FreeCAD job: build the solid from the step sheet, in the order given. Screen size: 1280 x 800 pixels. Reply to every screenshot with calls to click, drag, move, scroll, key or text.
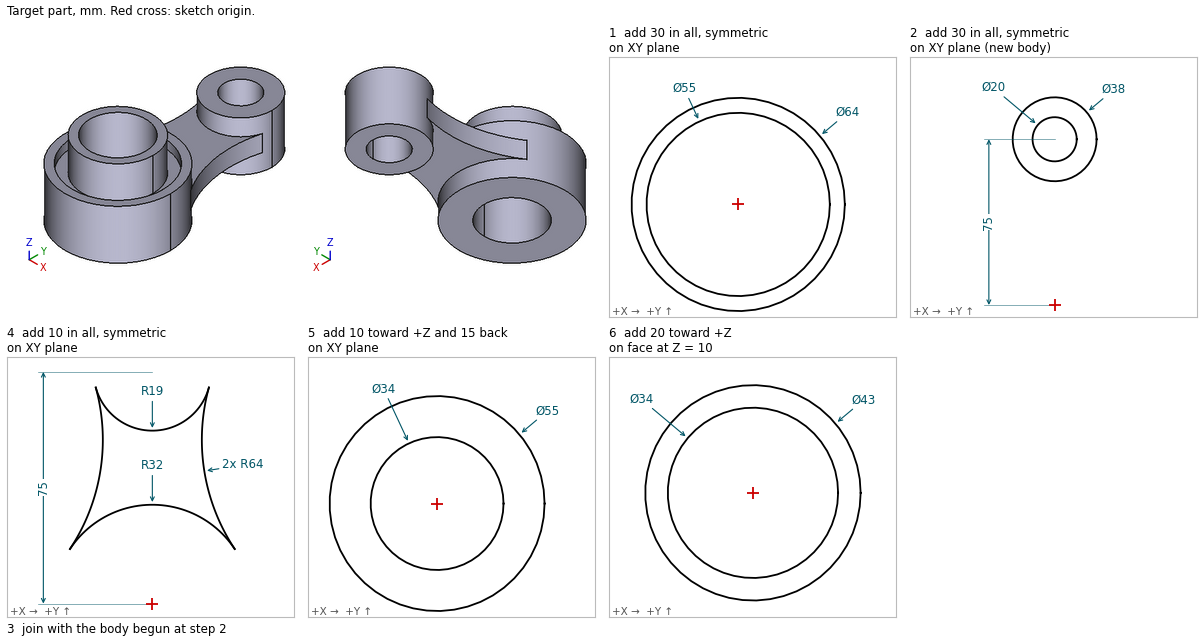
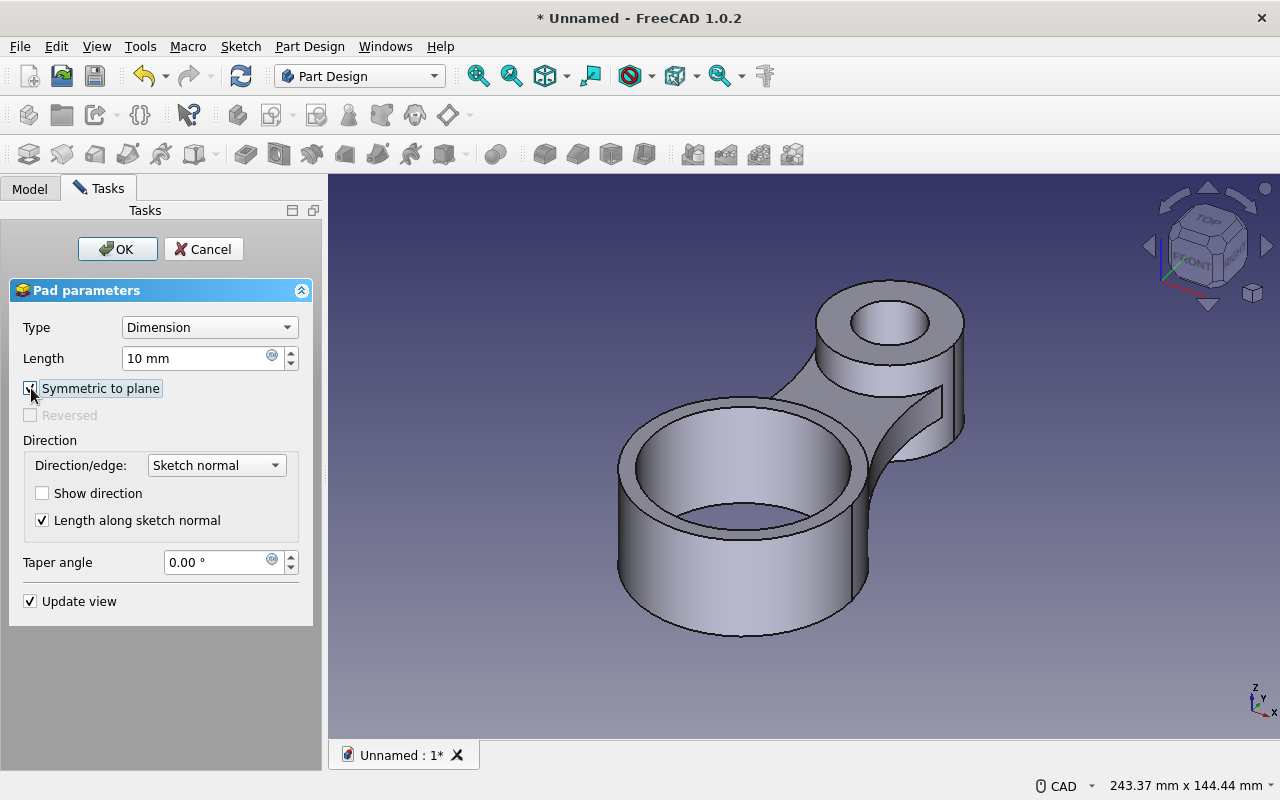
click(118, 249)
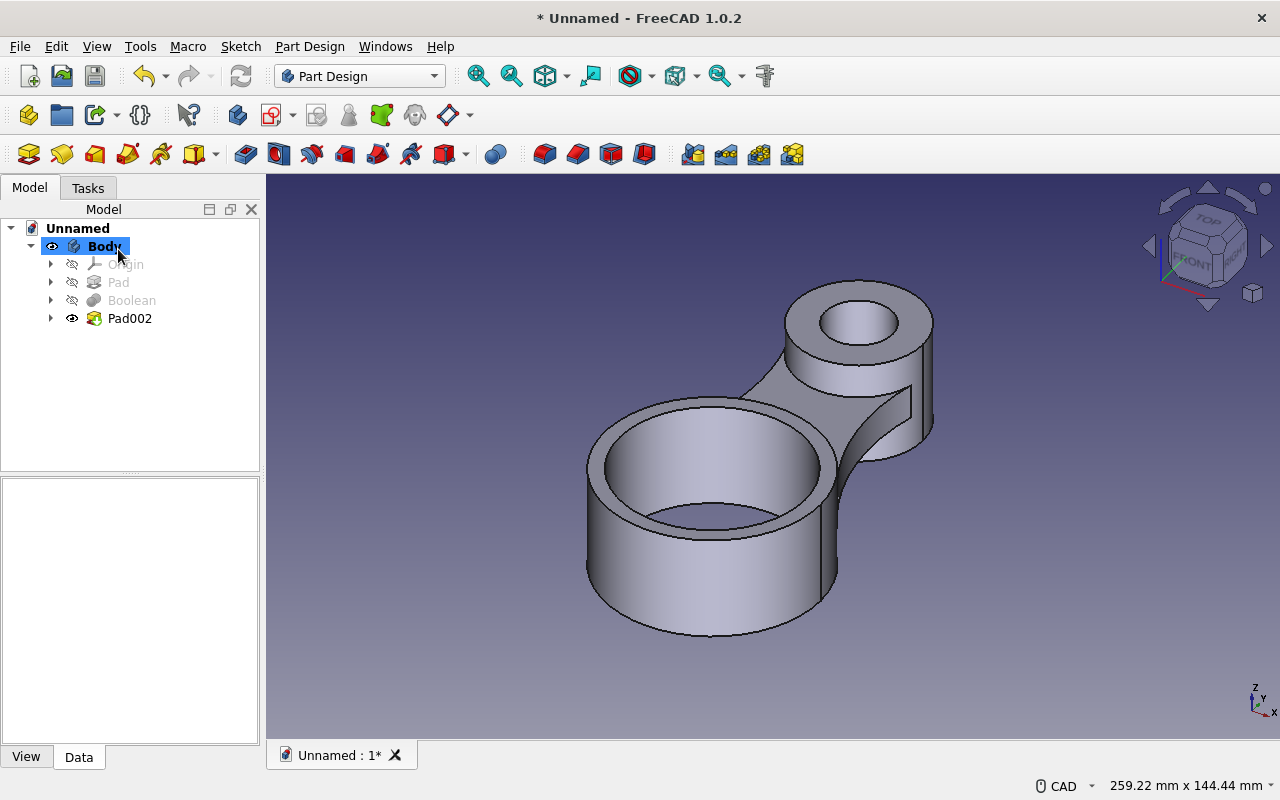
click(270, 116)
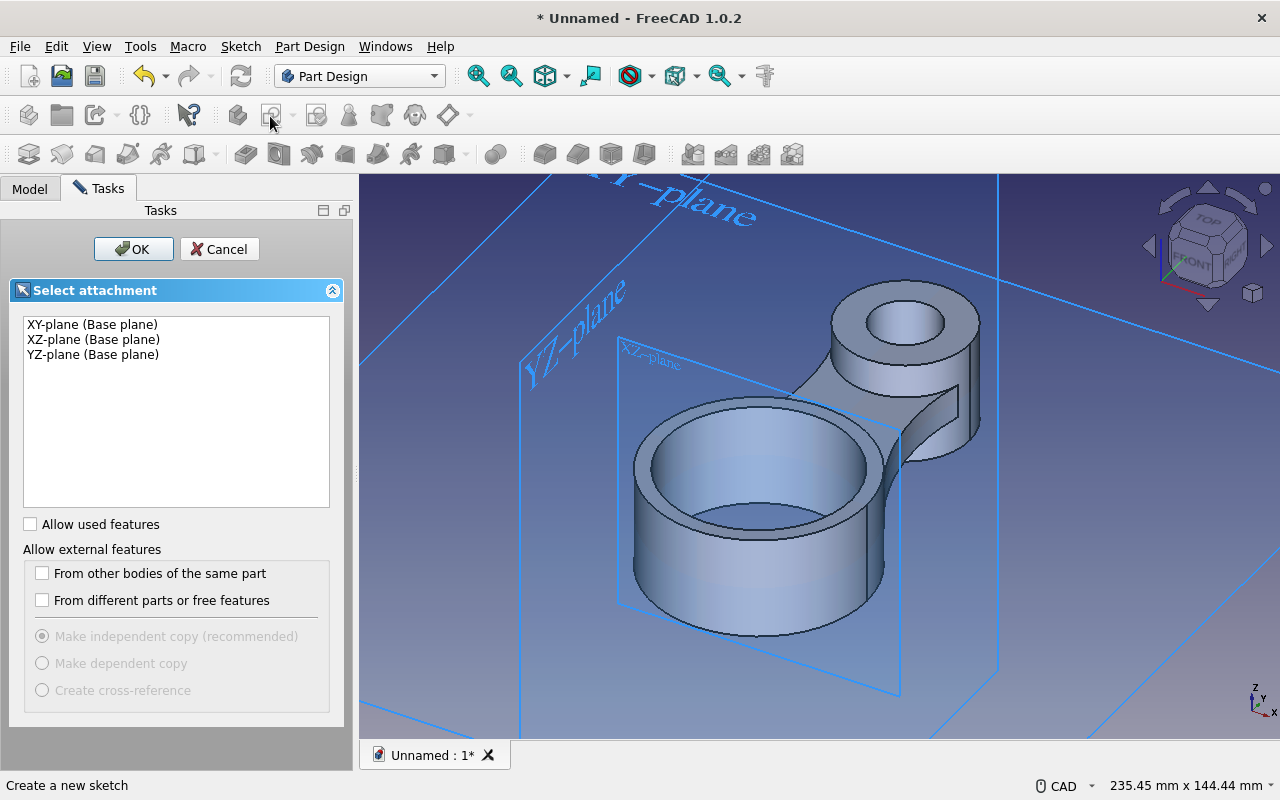
click(84, 324)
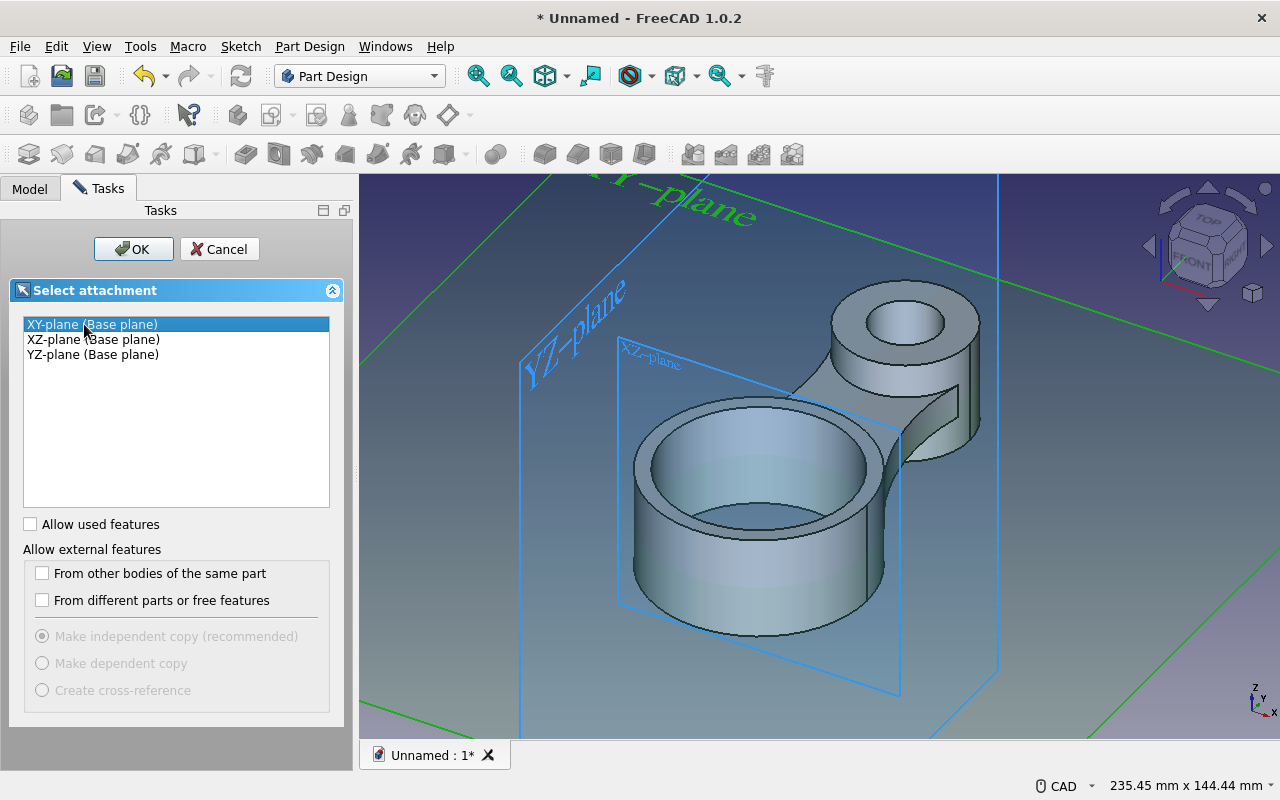
click(134, 249)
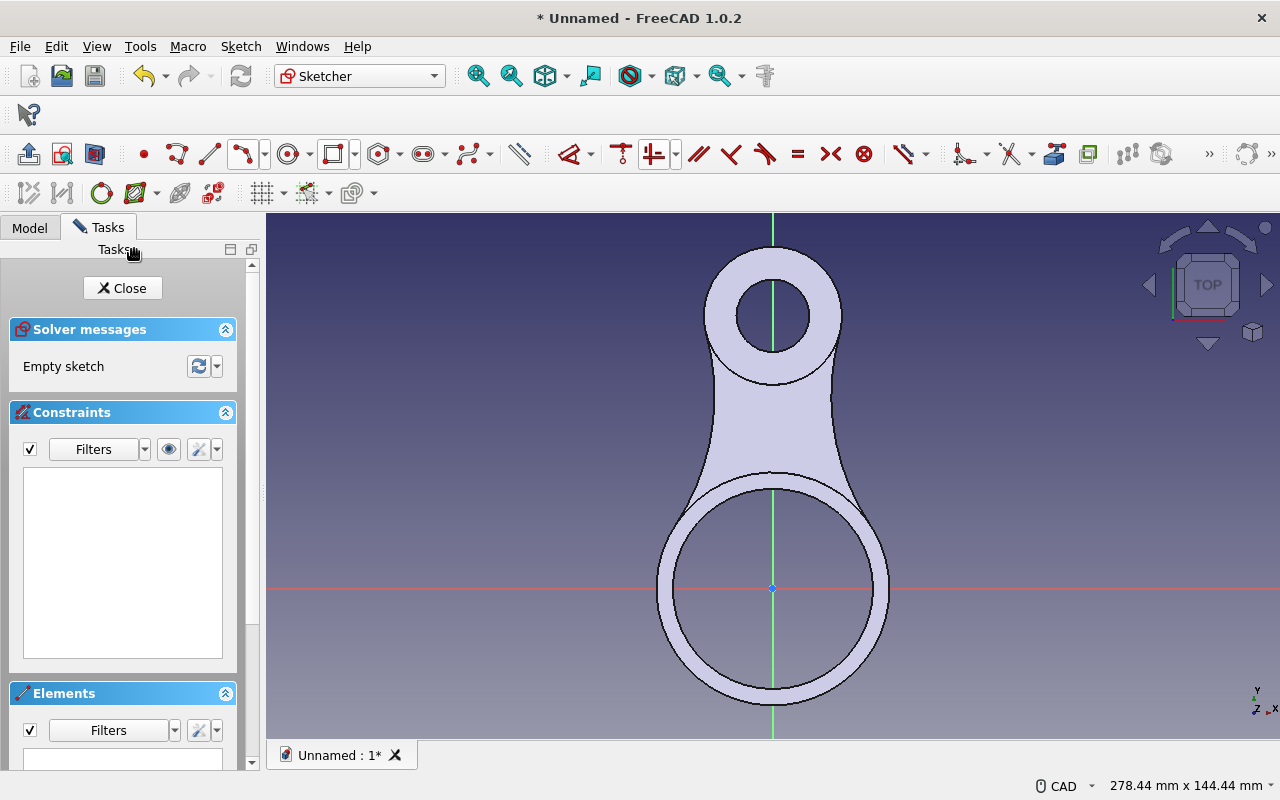
click(95, 154)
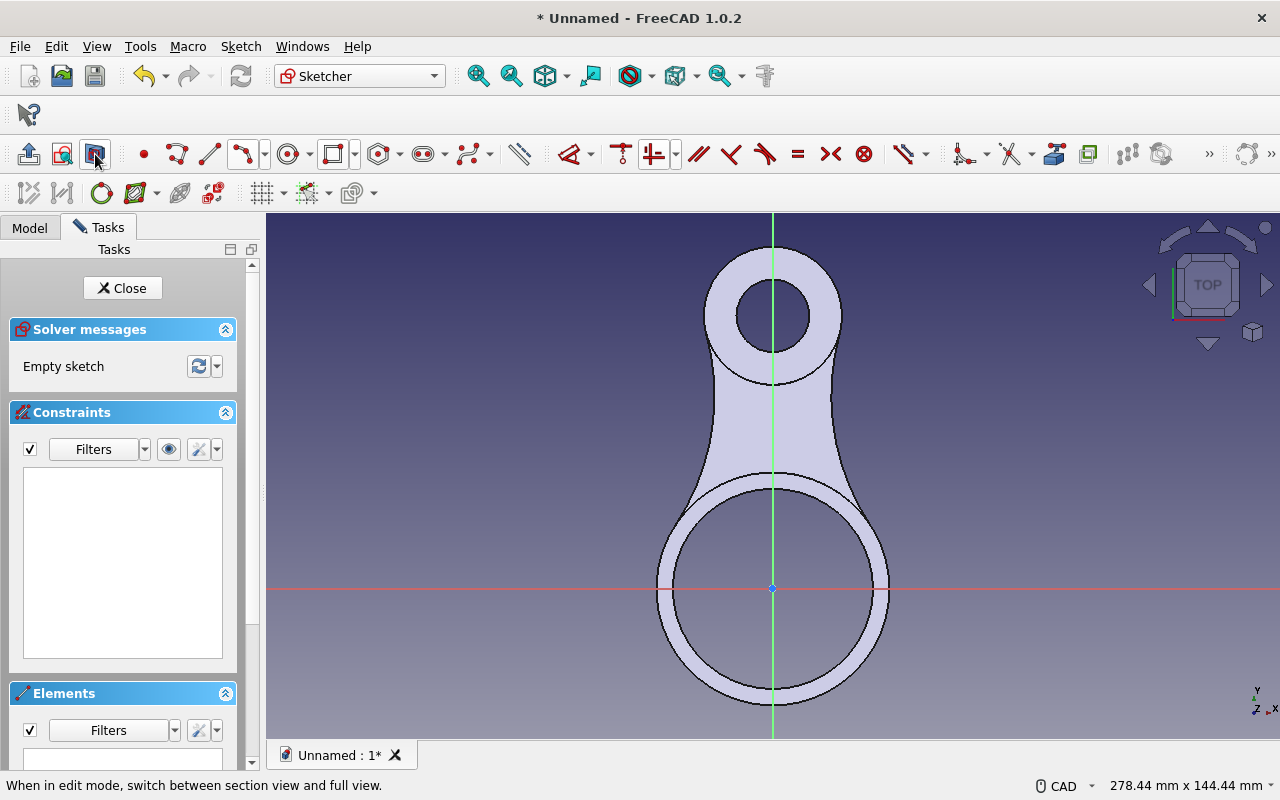
scroll(856, 711, up, 3)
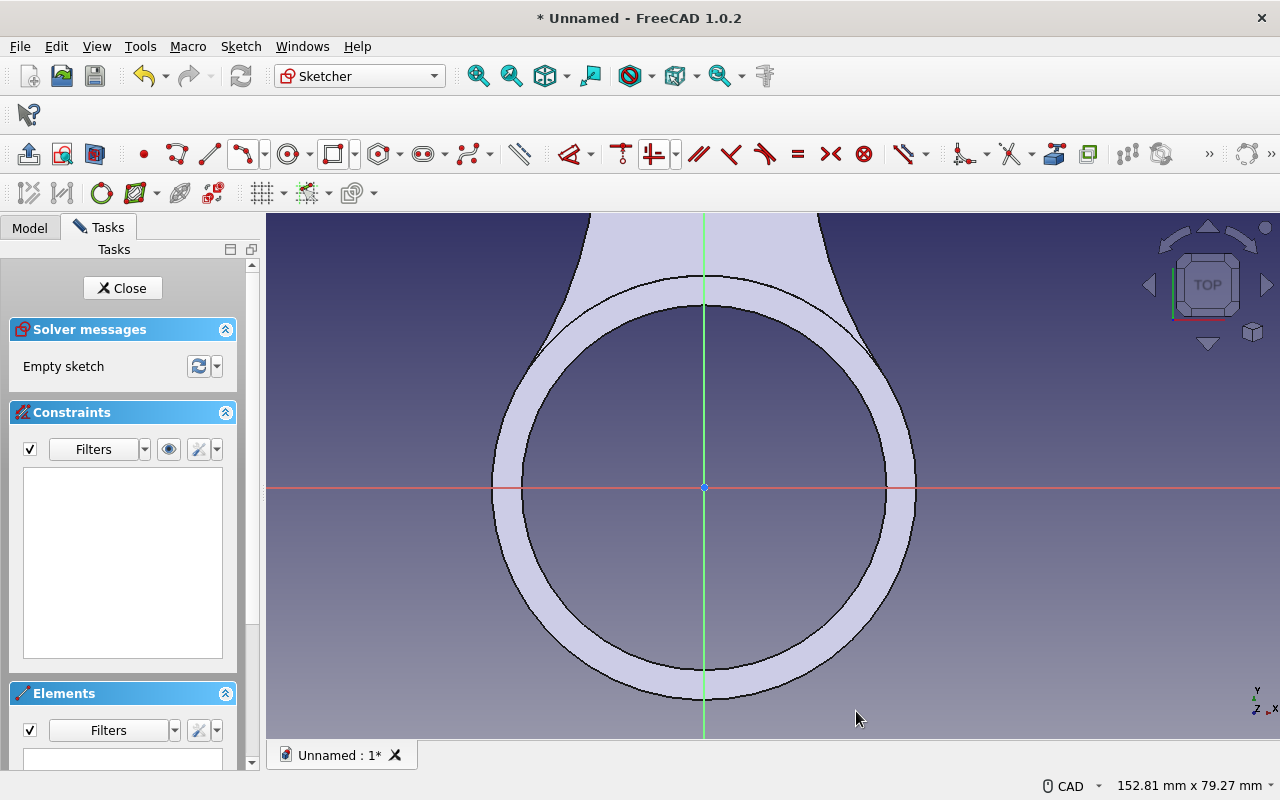
click(288, 154)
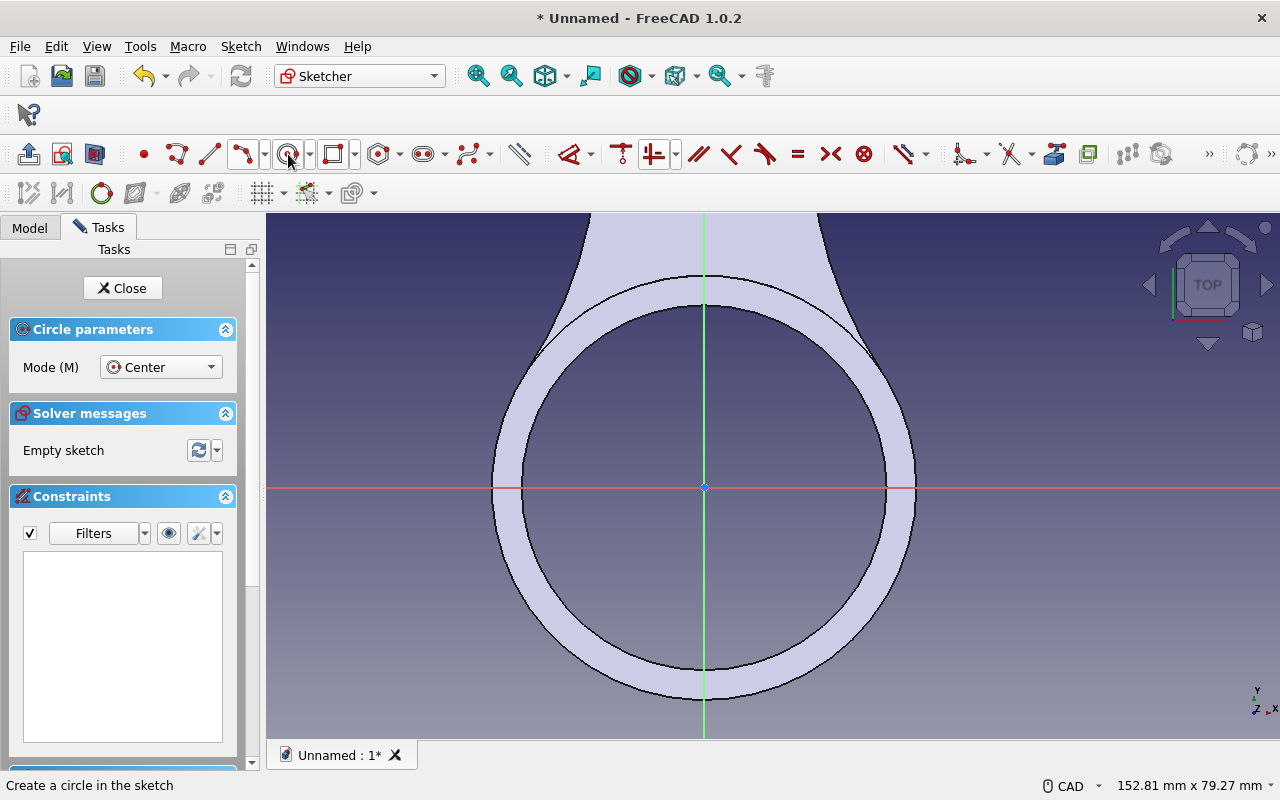
click(704, 488)
click(833, 359)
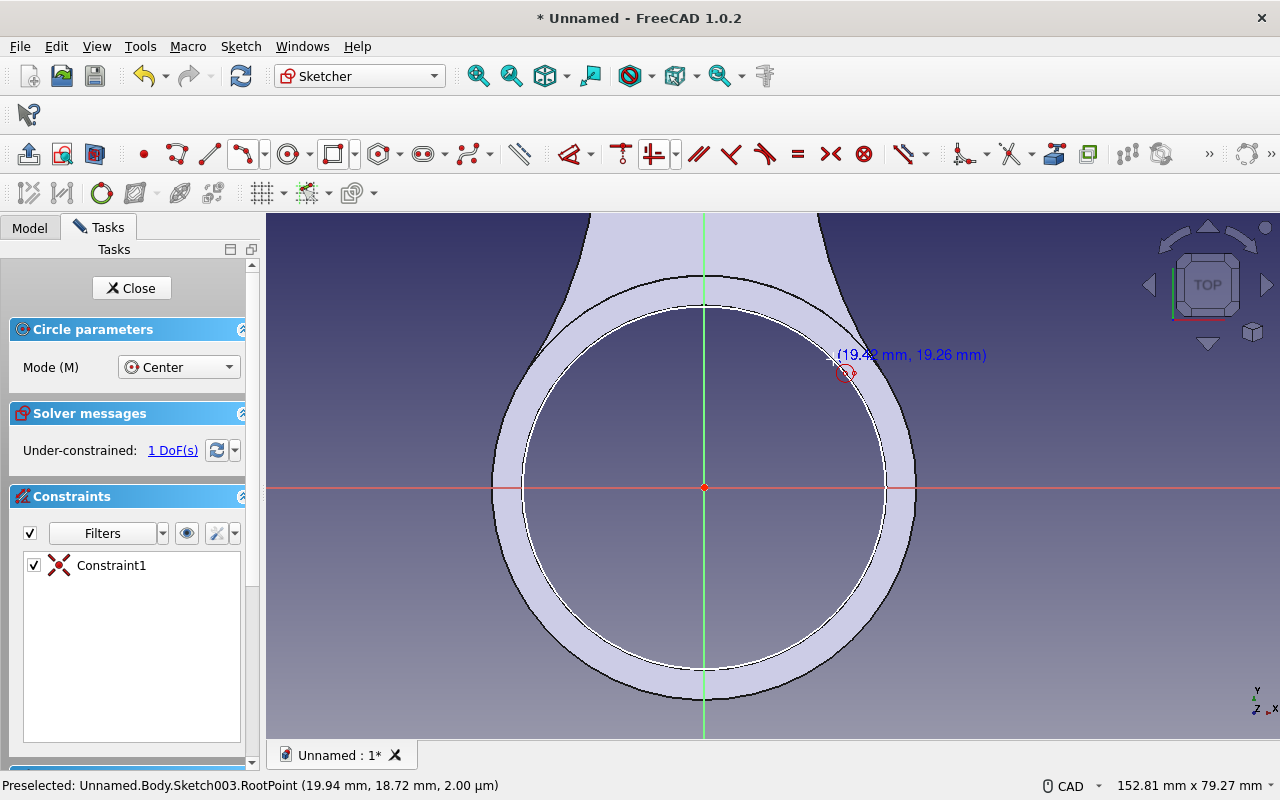
click(704, 488)
click(784, 408)
key(Escape)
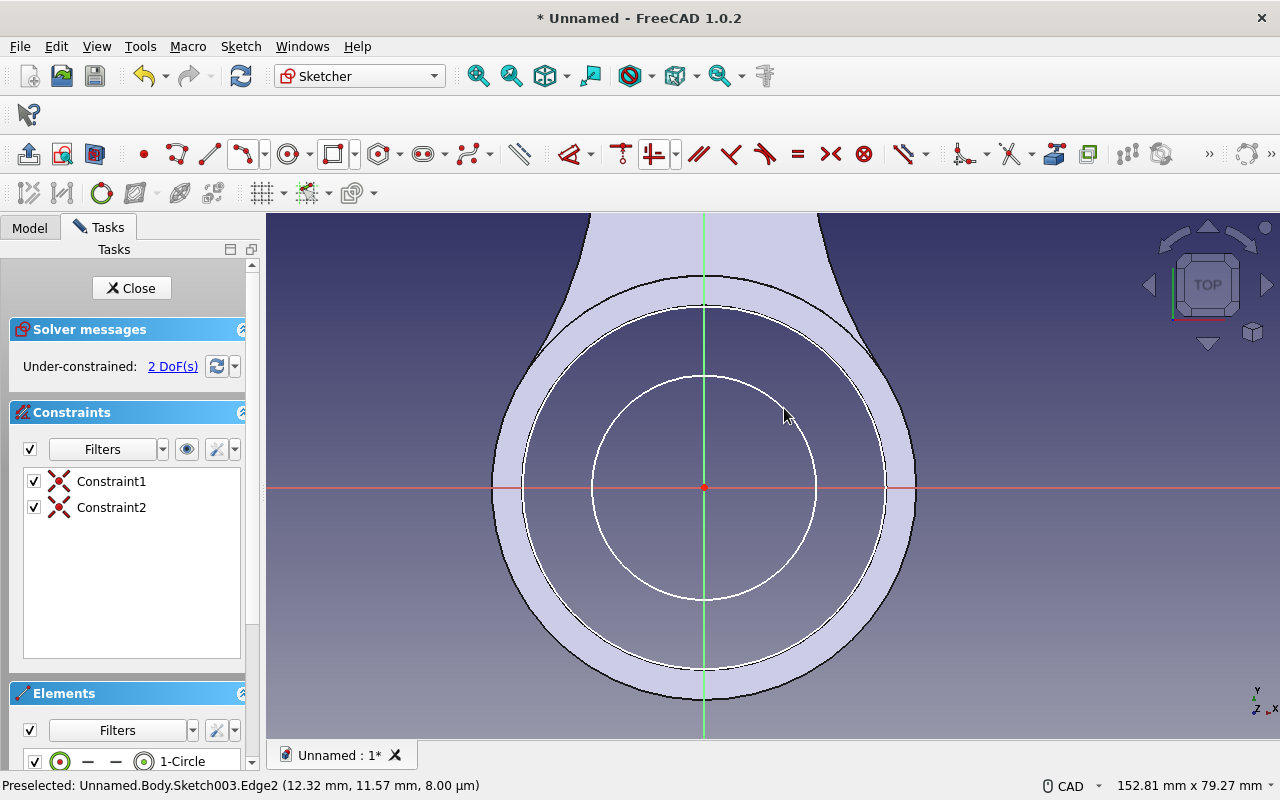
key(d)